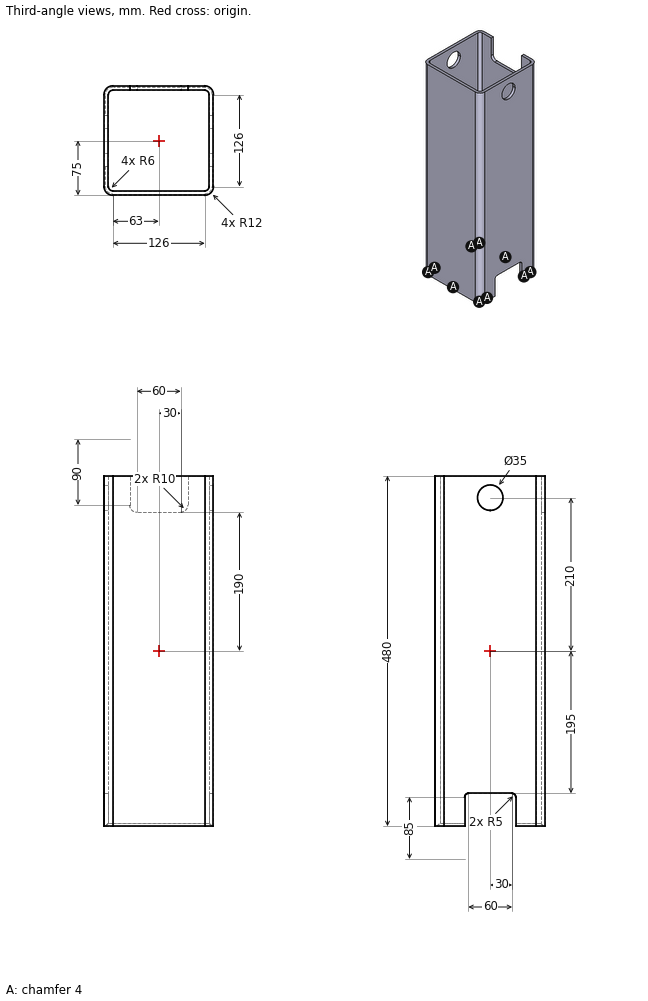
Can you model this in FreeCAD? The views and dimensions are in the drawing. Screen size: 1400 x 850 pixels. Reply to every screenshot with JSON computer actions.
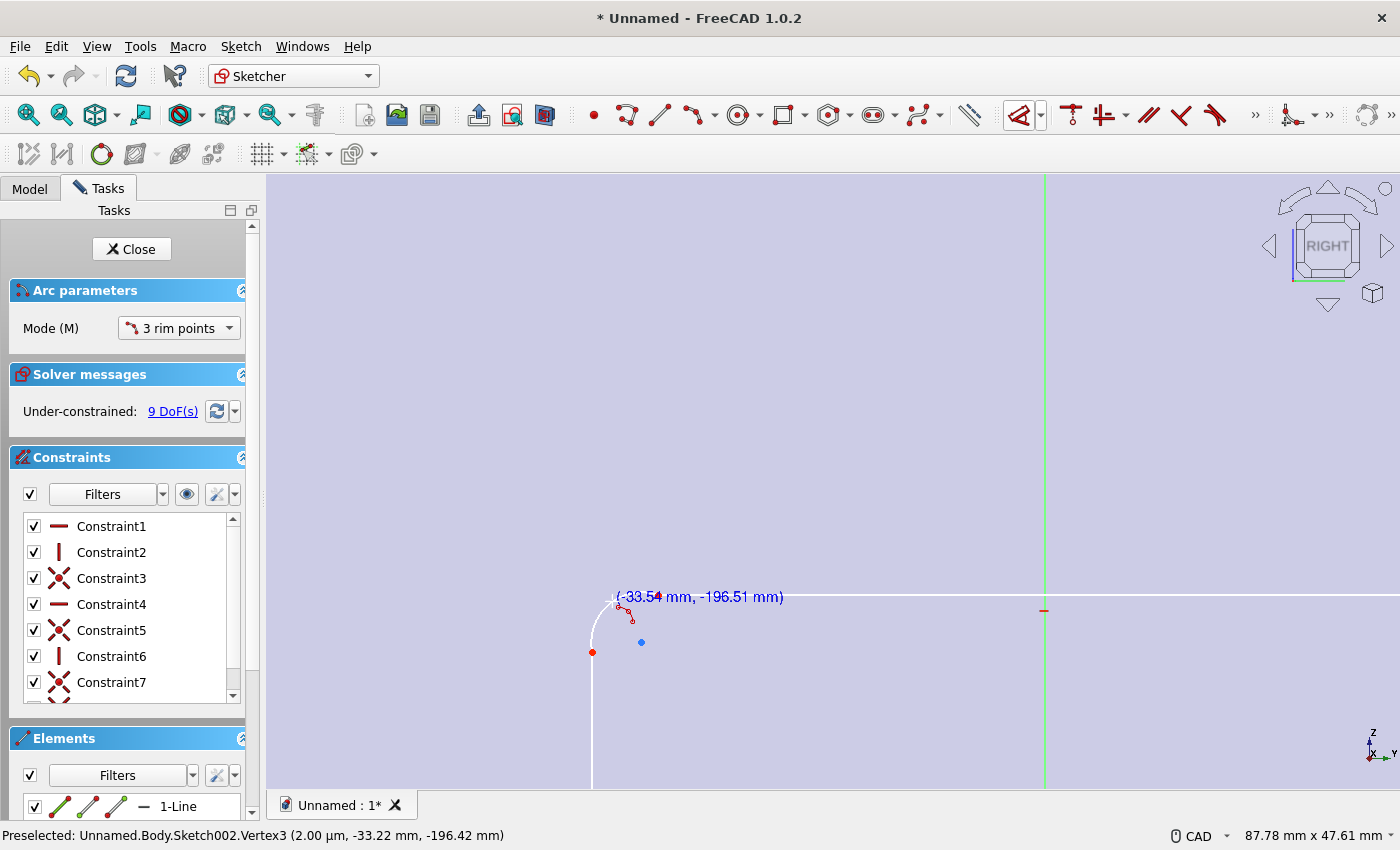
{"action": "scroll", "coordinate": [746, 614], "scroll_direction": "down", "scroll_amount": 14}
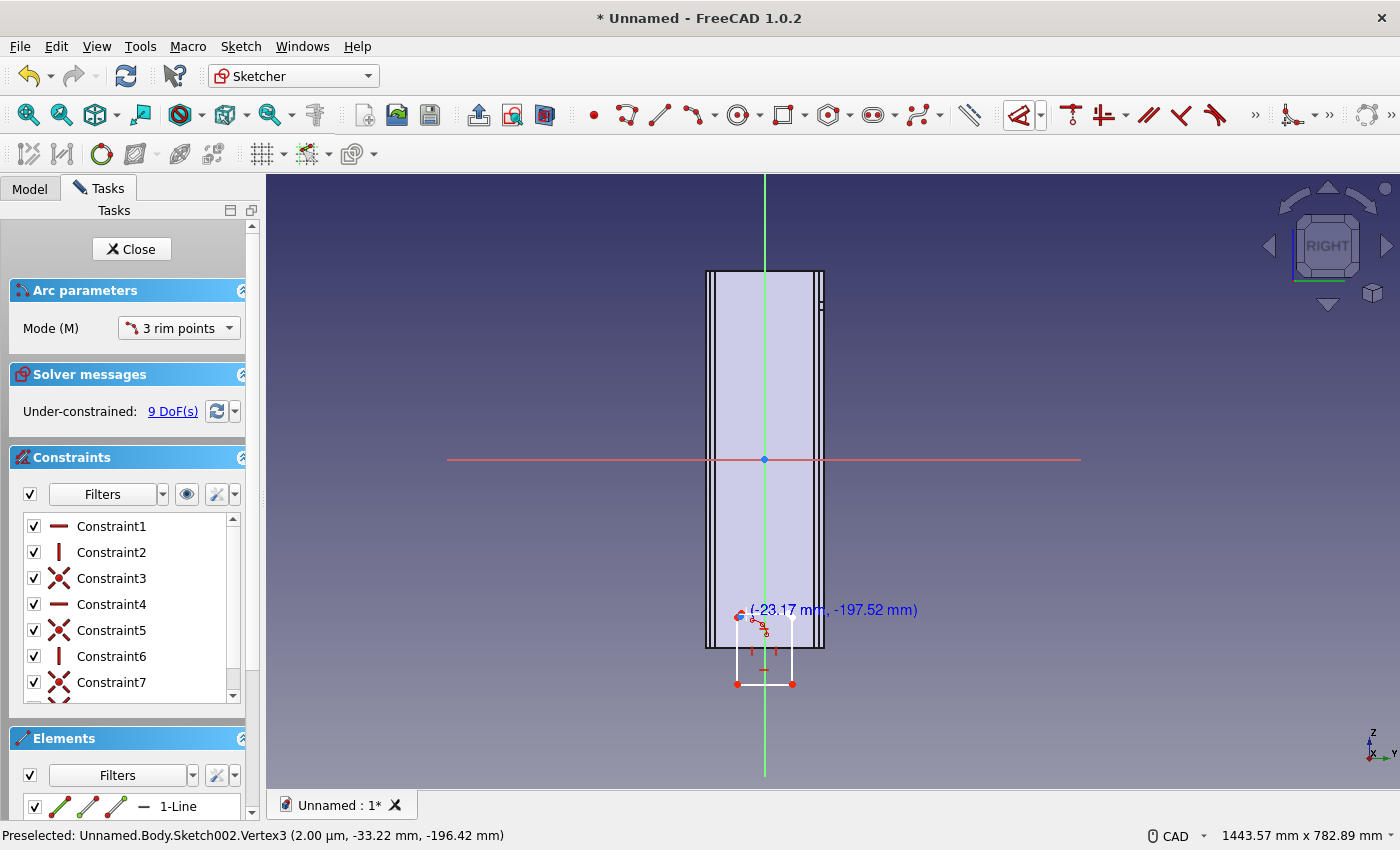
{"action": "scroll", "coordinate": [792, 617], "scroll_direction": "up", "scroll_amount": 6}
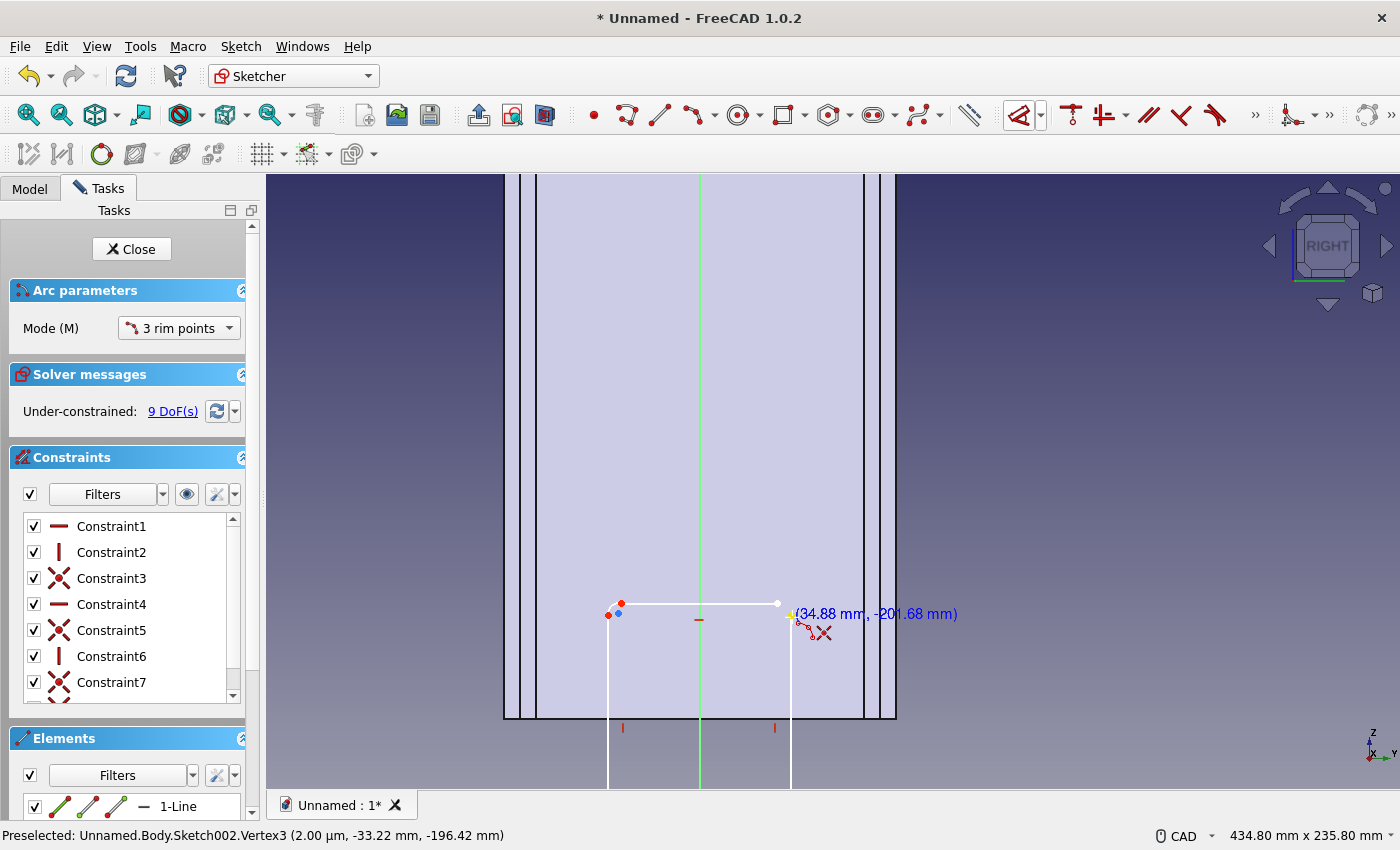
{"action": "left_click", "coordinate": [791, 615]}
{"action": "left_click", "coordinate": [778, 604]}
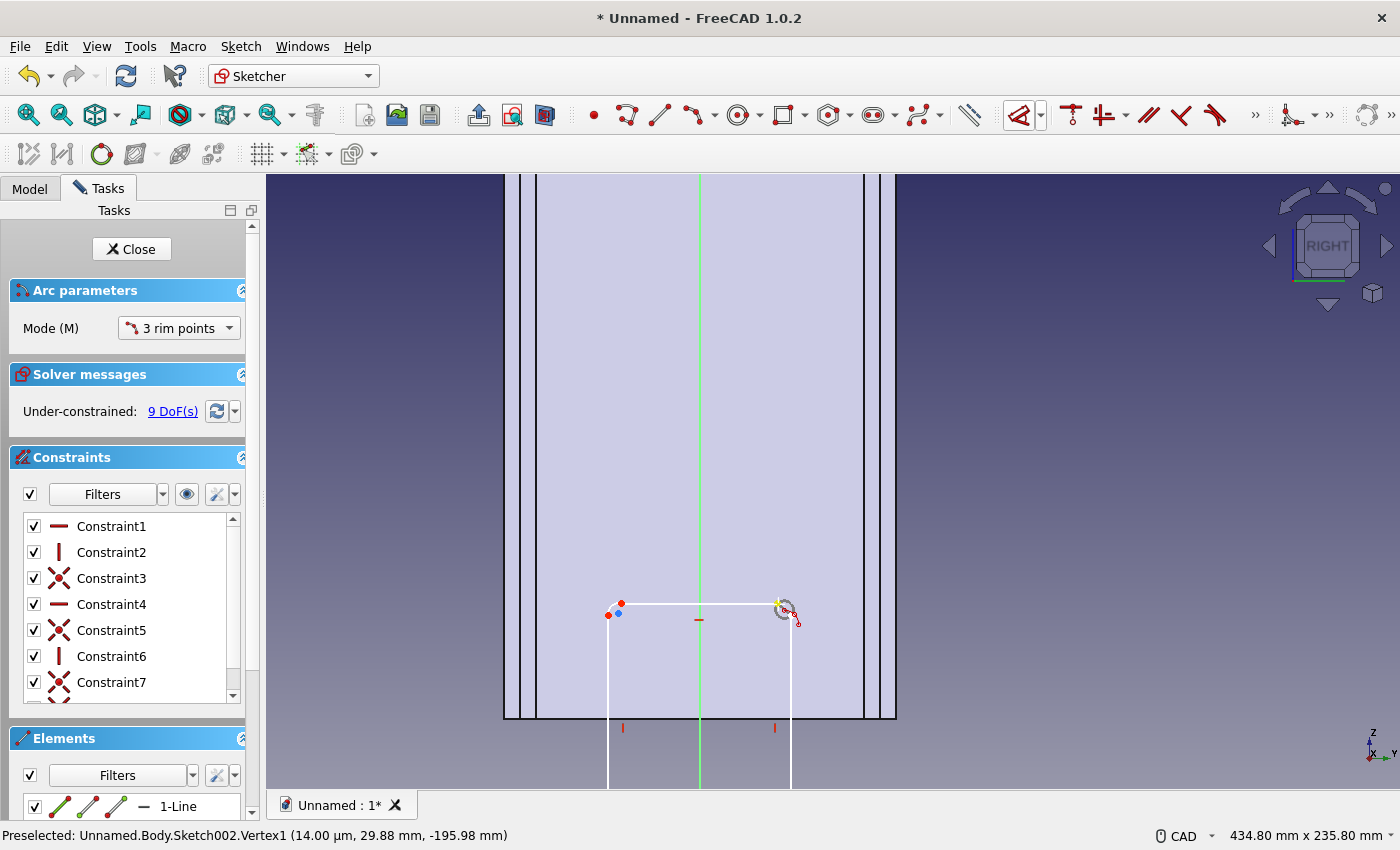
{"action": "scroll", "coordinate": [787, 605], "scroll_direction": "up", "scroll_amount": 8}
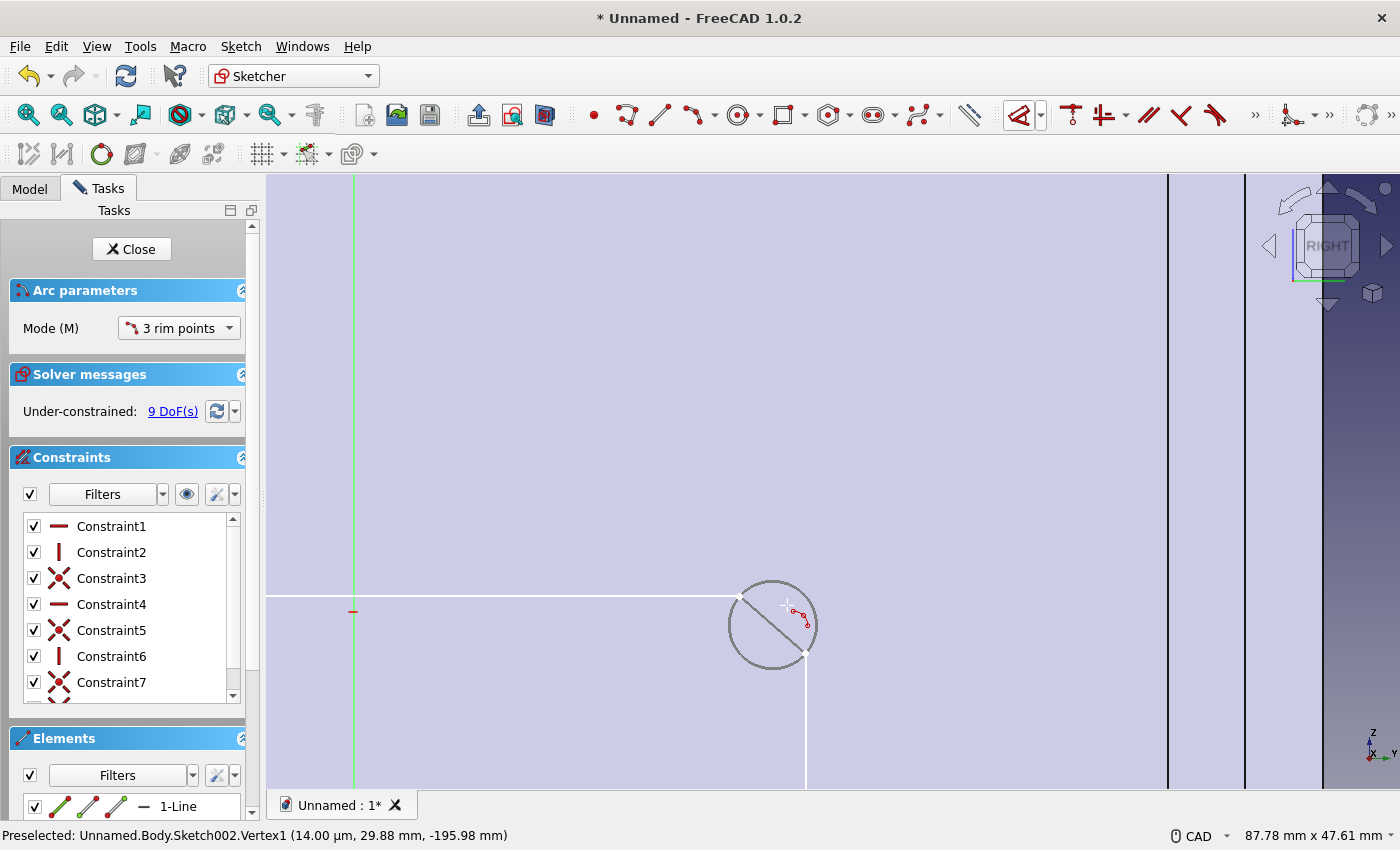
{"action": "left_click", "coordinate": [787, 602]}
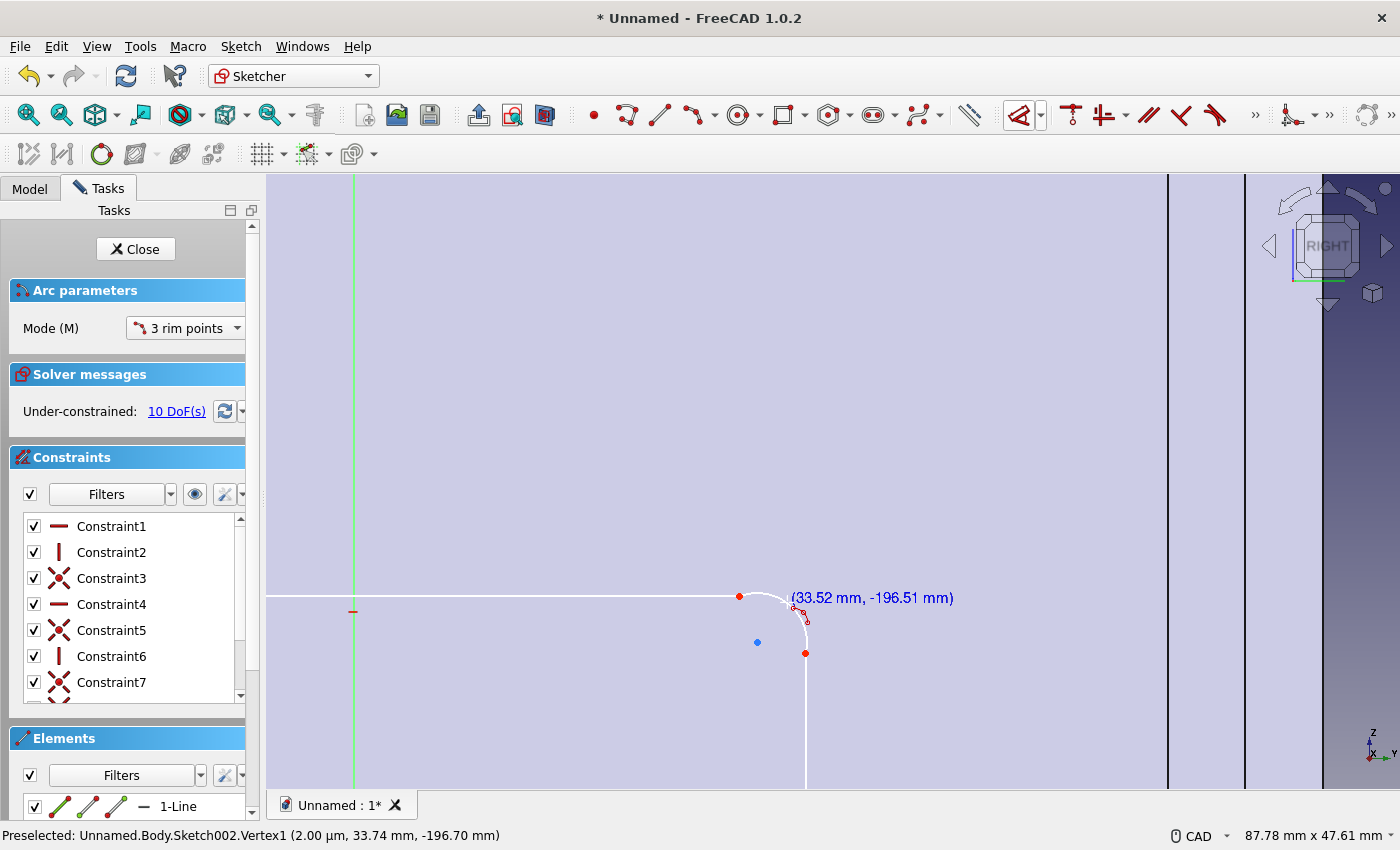
{"action": "key", "text": "g c"}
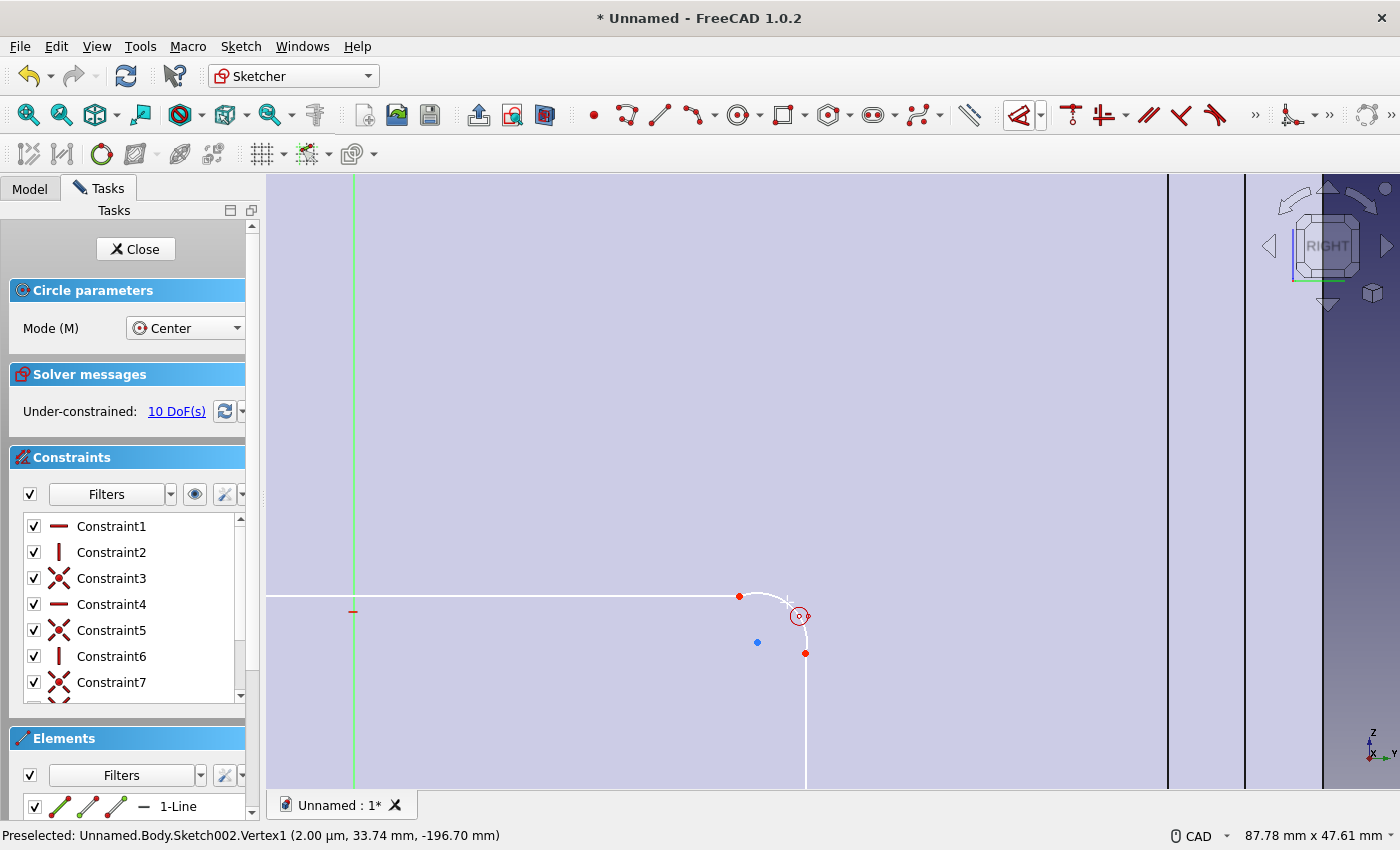
{"action": "scroll", "coordinate": [791, 614], "scroll_direction": "down", "scroll_amount": 14}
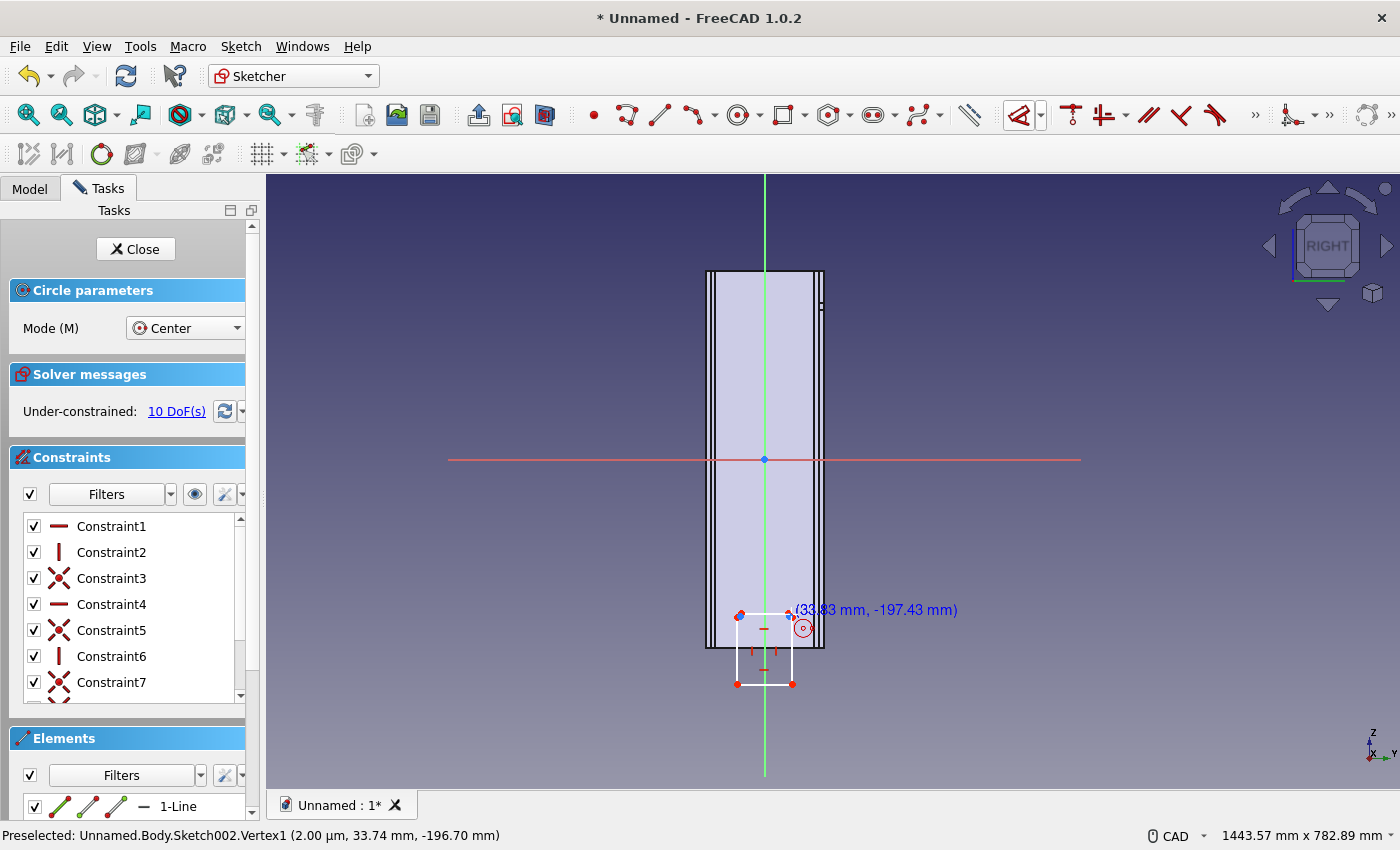
{"action": "scroll", "coordinate": [765, 295], "scroll_direction": "up", "scroll_amount": 3}